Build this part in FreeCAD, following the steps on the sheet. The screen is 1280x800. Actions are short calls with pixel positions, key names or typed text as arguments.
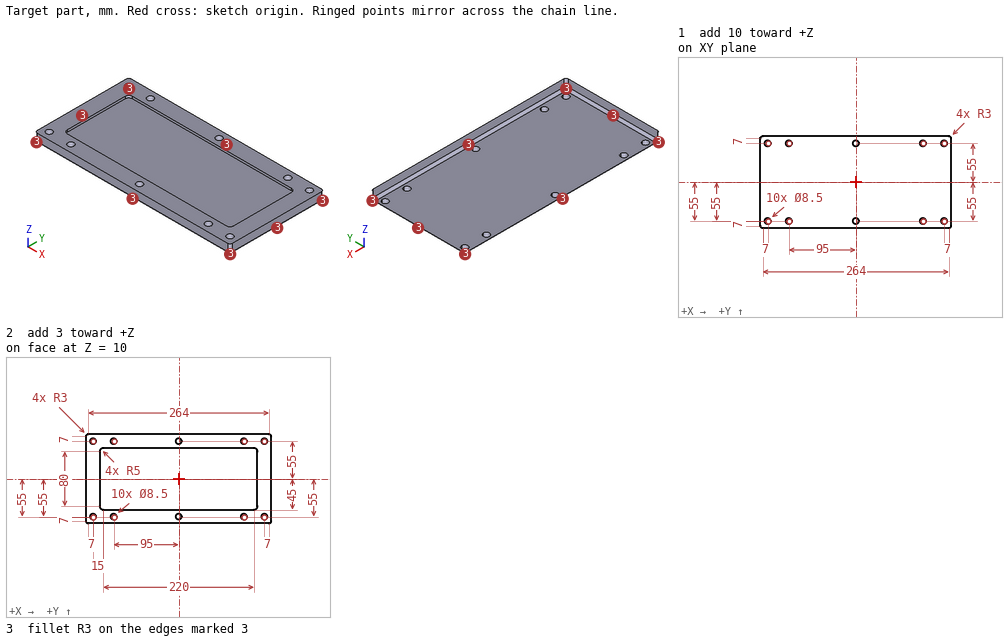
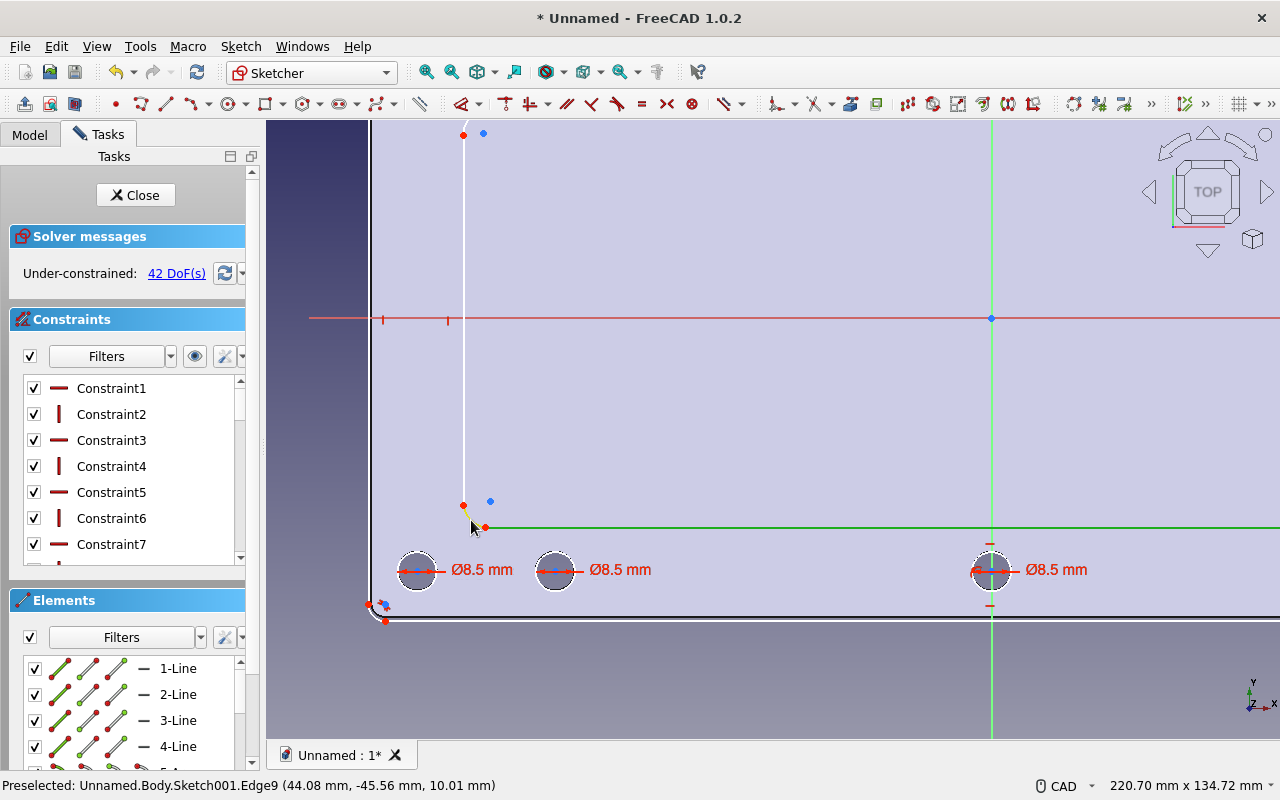
click(471, 520)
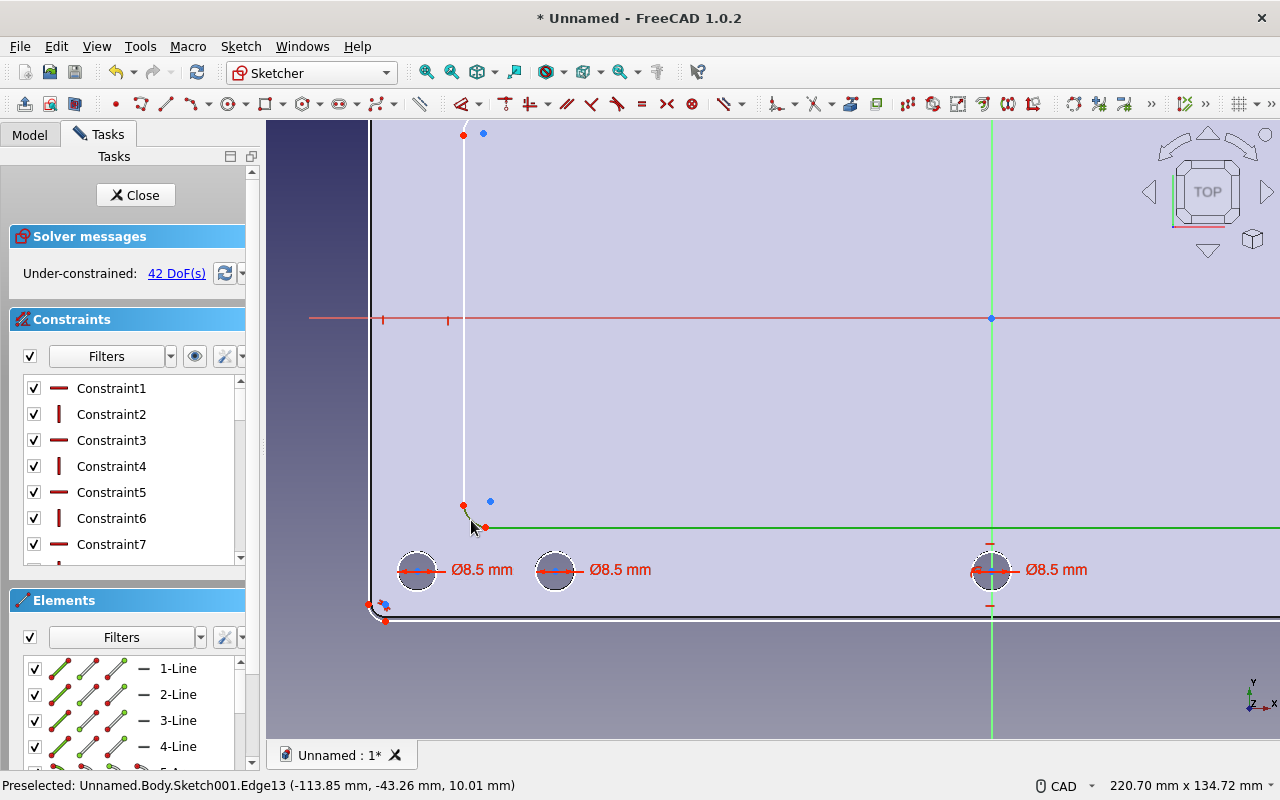
click(617, 104)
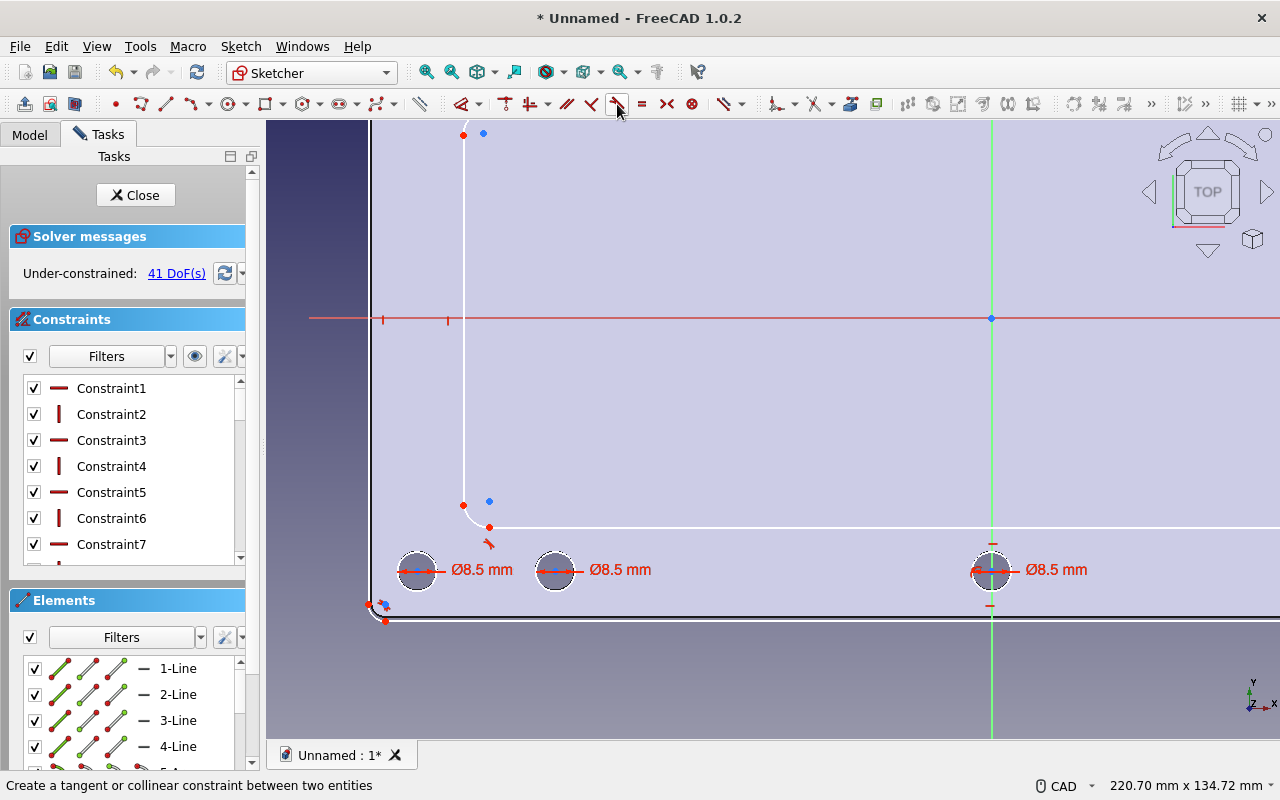
click(792, 528)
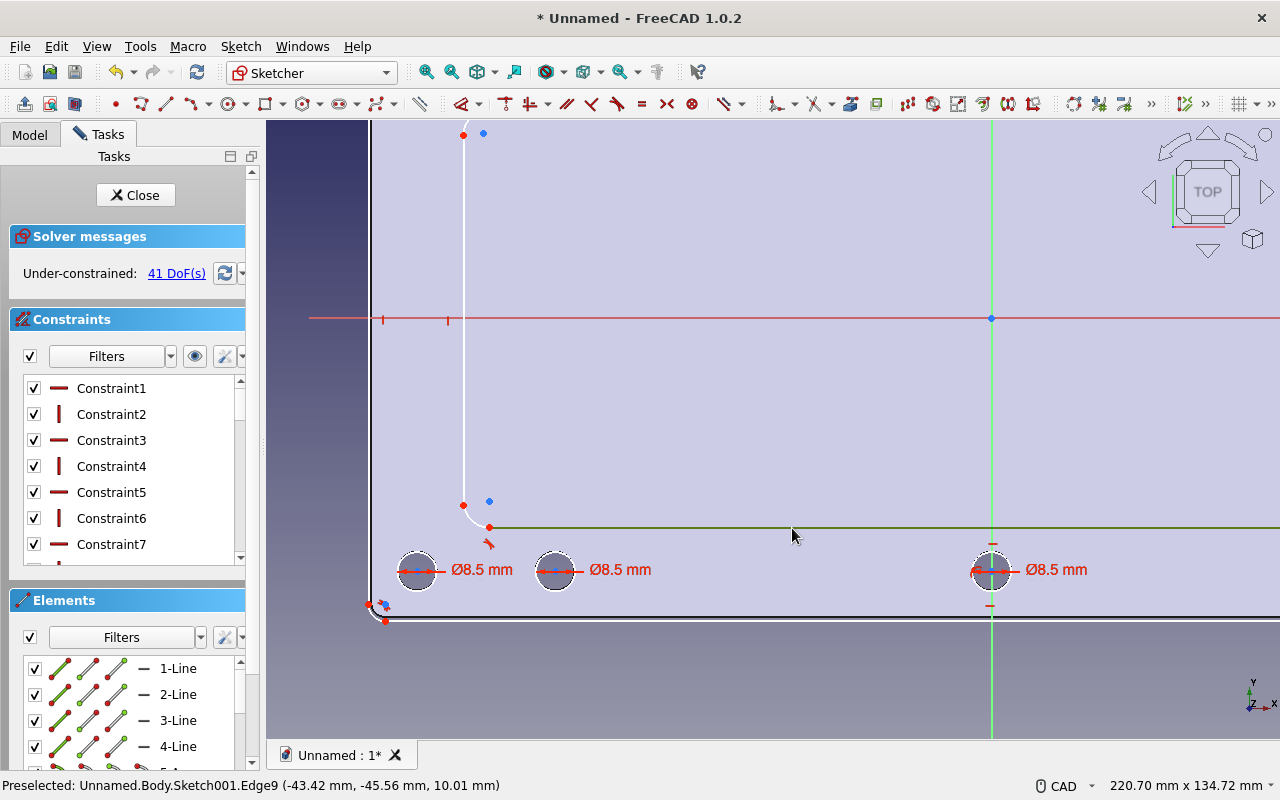
scroll(470, 520, down, 4)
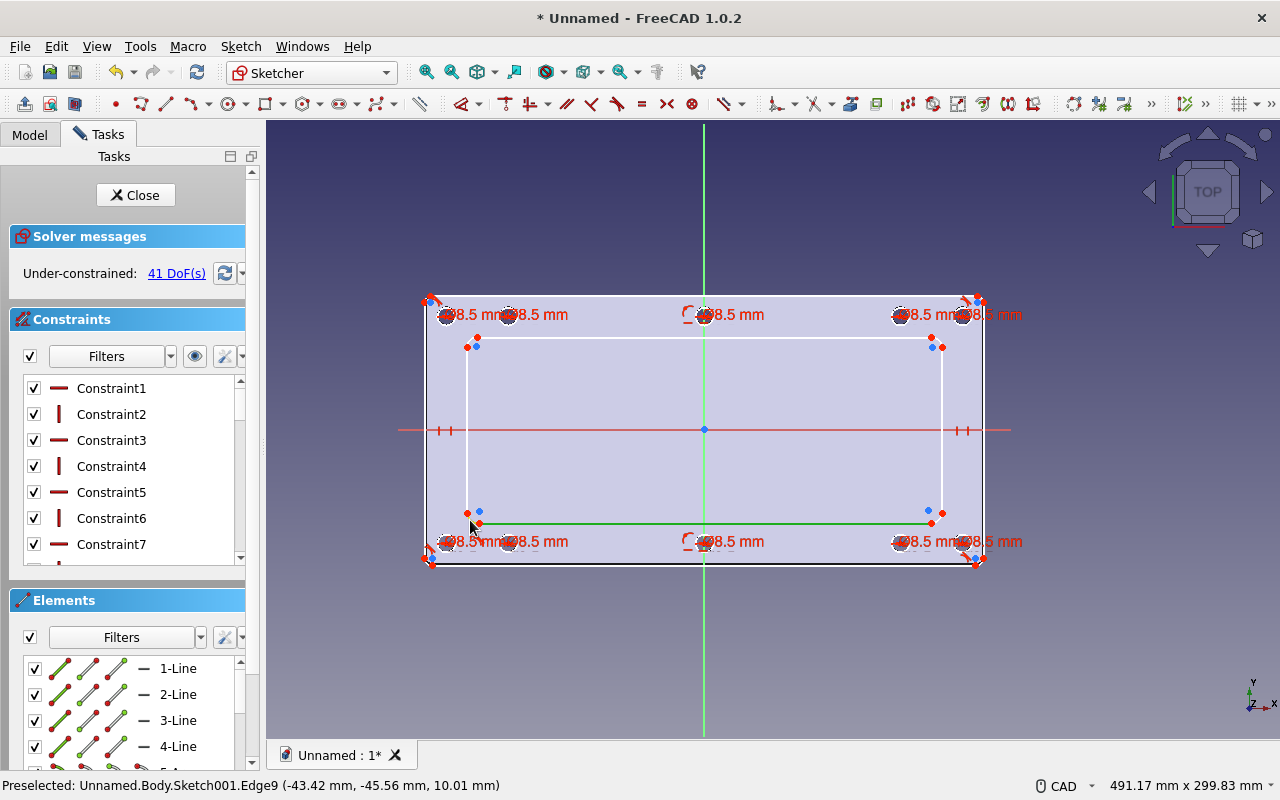
scroll(936, 522, up, 6)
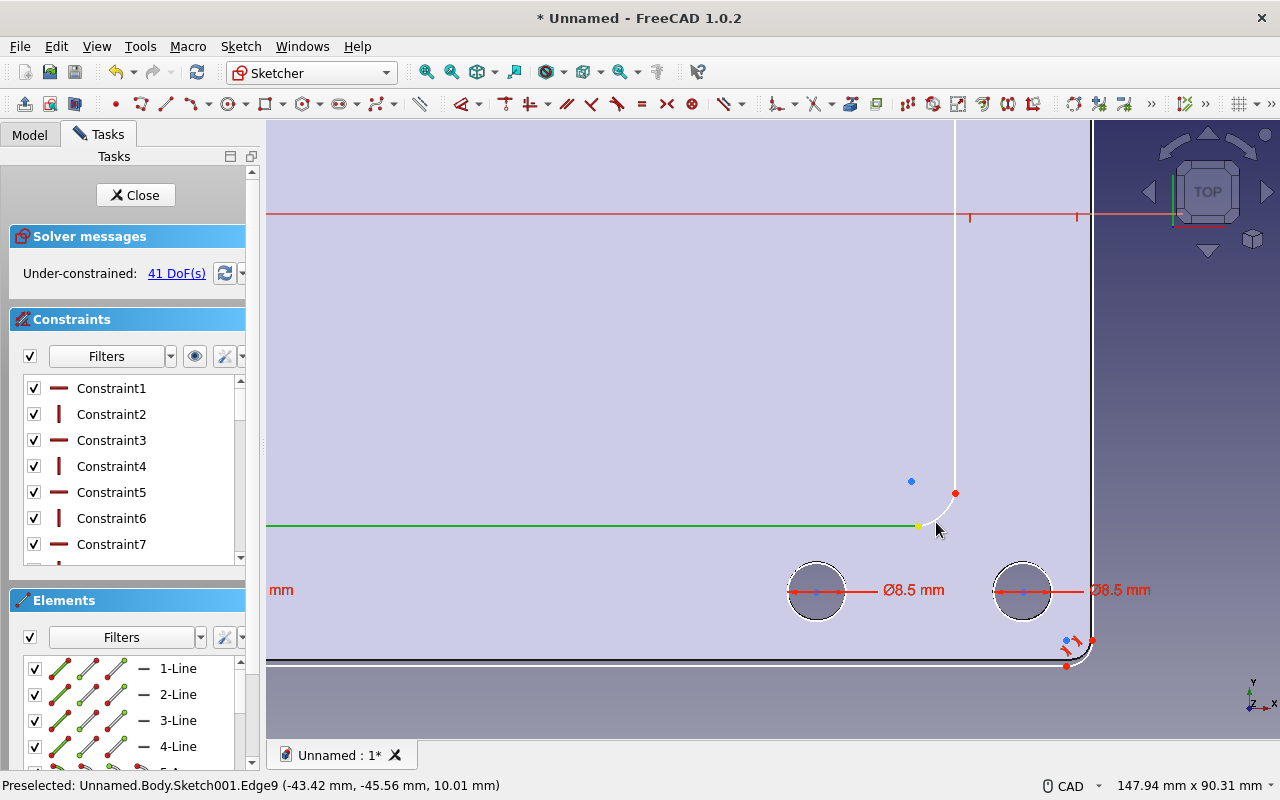
click(933, 521)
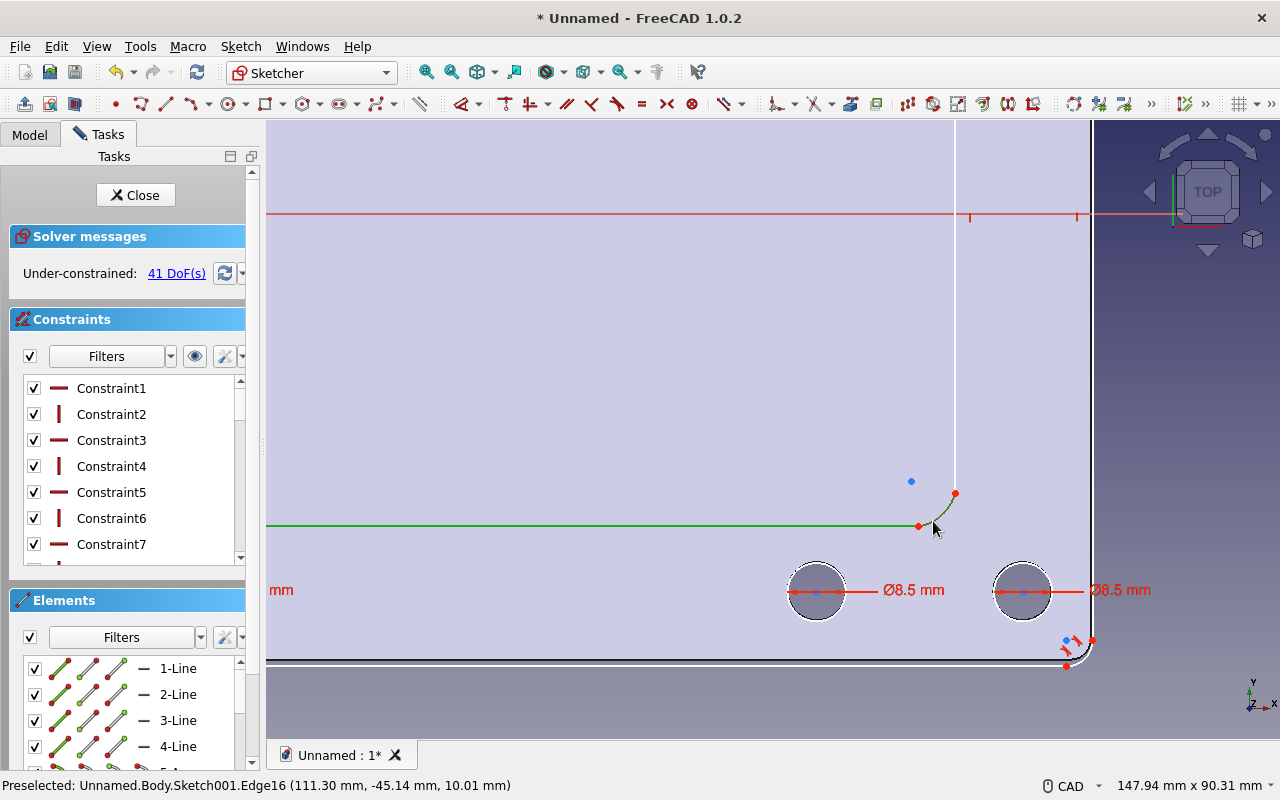
click(617, 104)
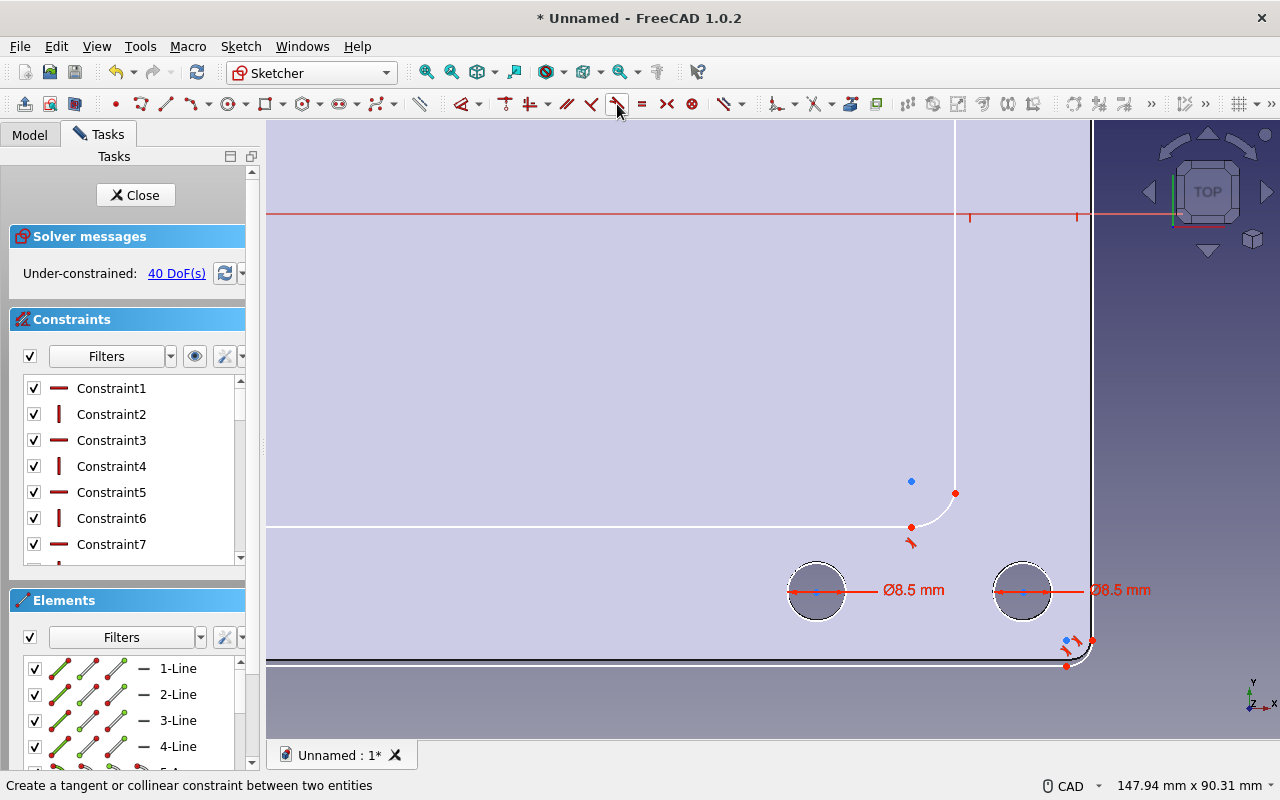
scroll(937, 522, down, 6)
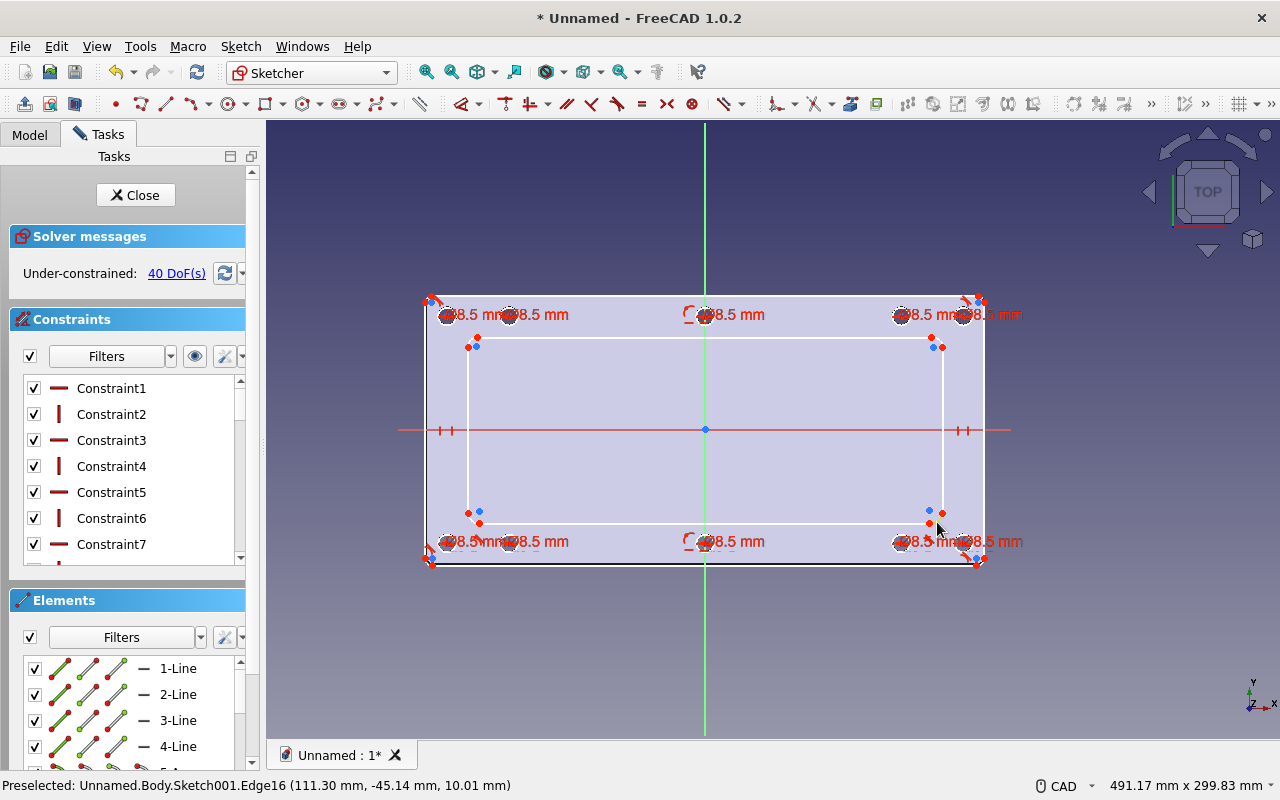
click(468, 464)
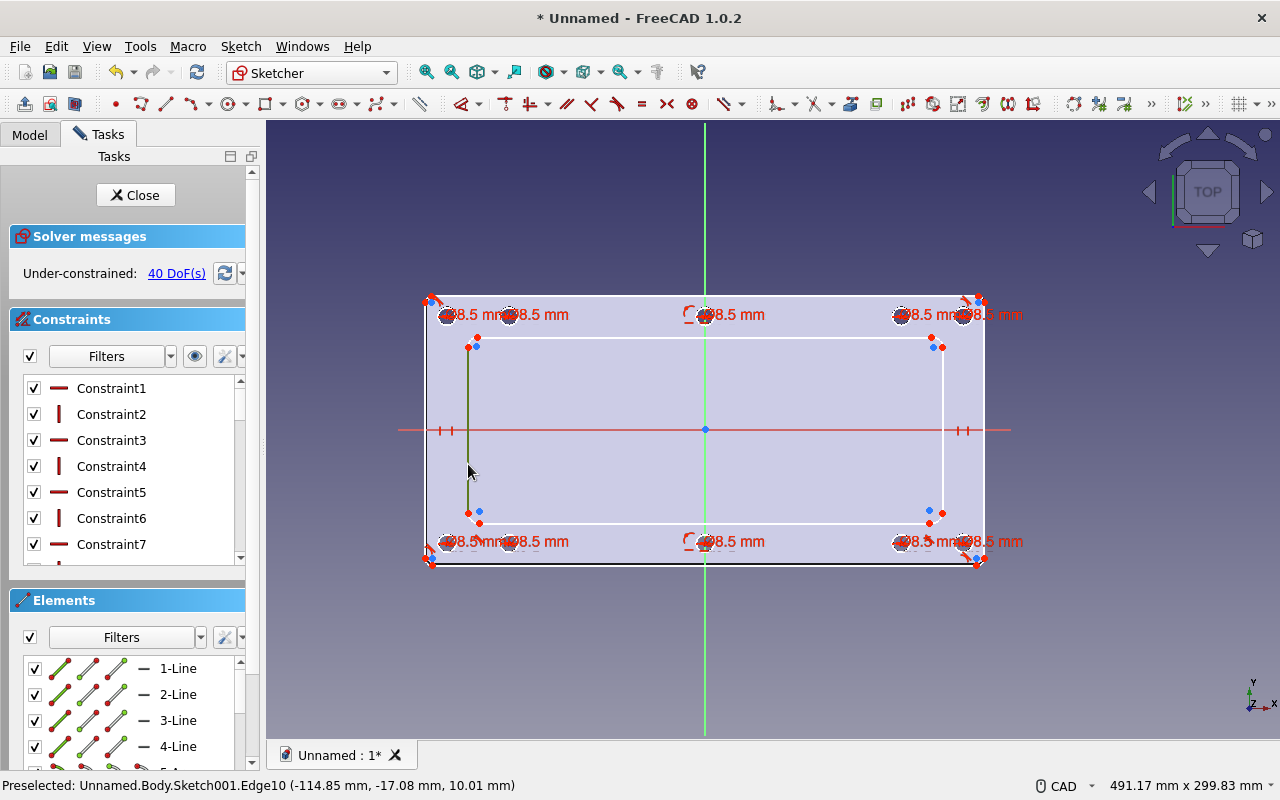
scroll(472, 521, up, 3)